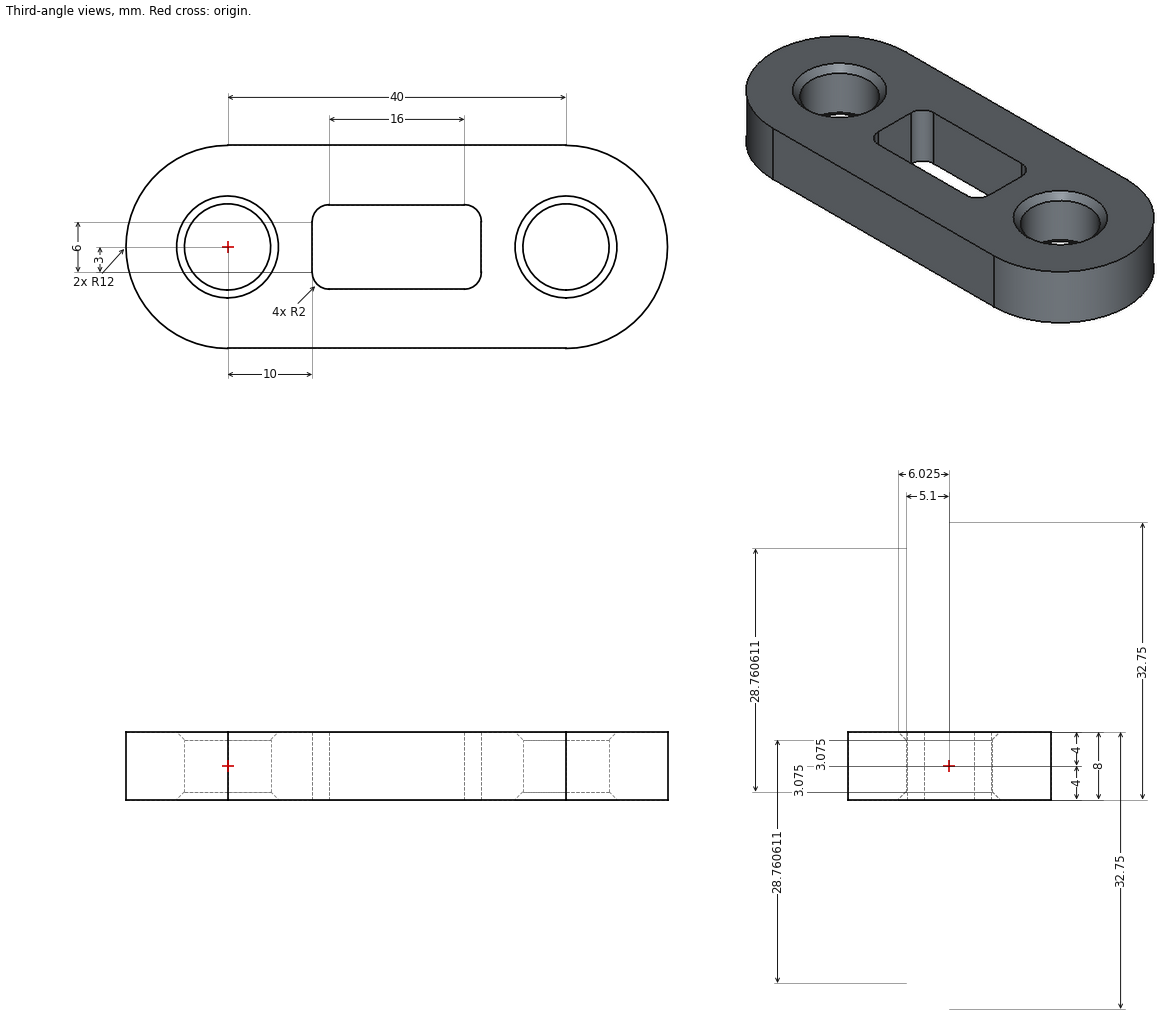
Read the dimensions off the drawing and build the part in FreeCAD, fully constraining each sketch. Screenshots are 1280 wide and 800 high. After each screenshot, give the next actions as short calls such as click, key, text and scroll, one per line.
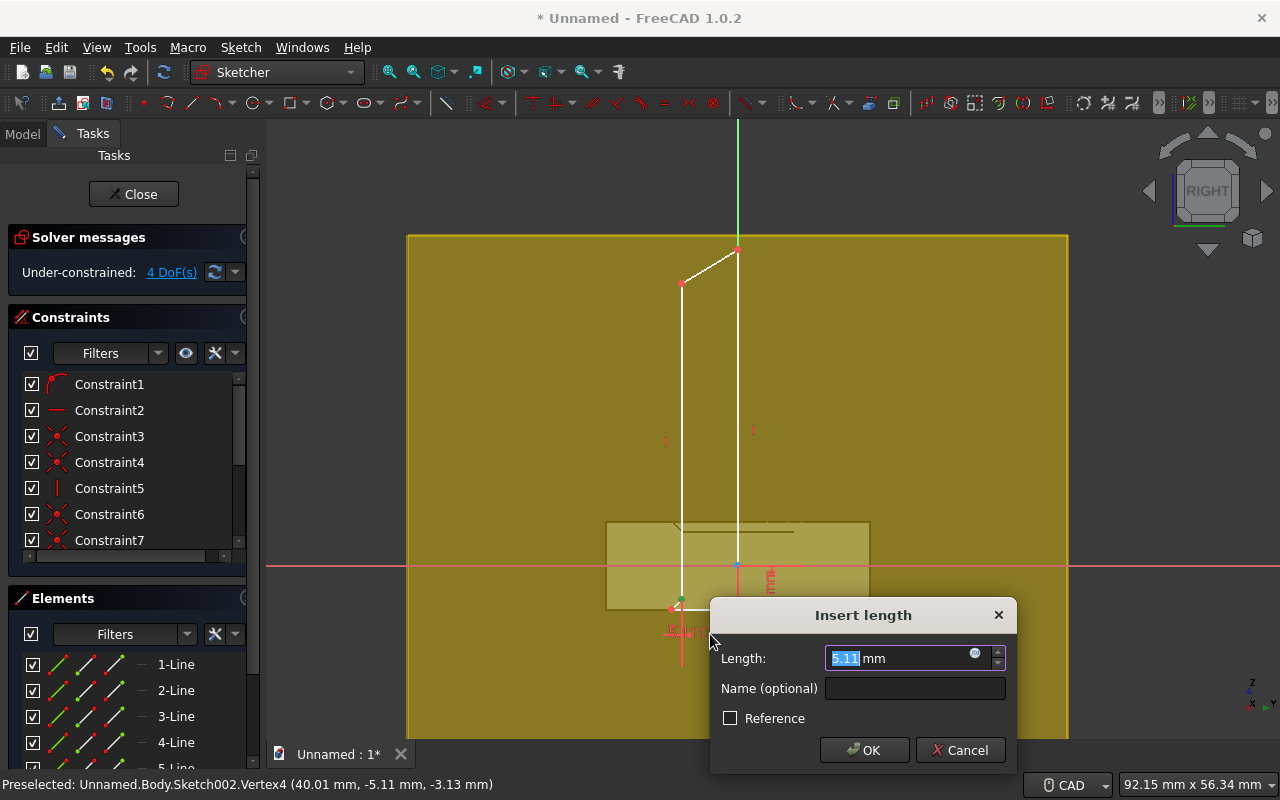
text(5.1)
key(Return)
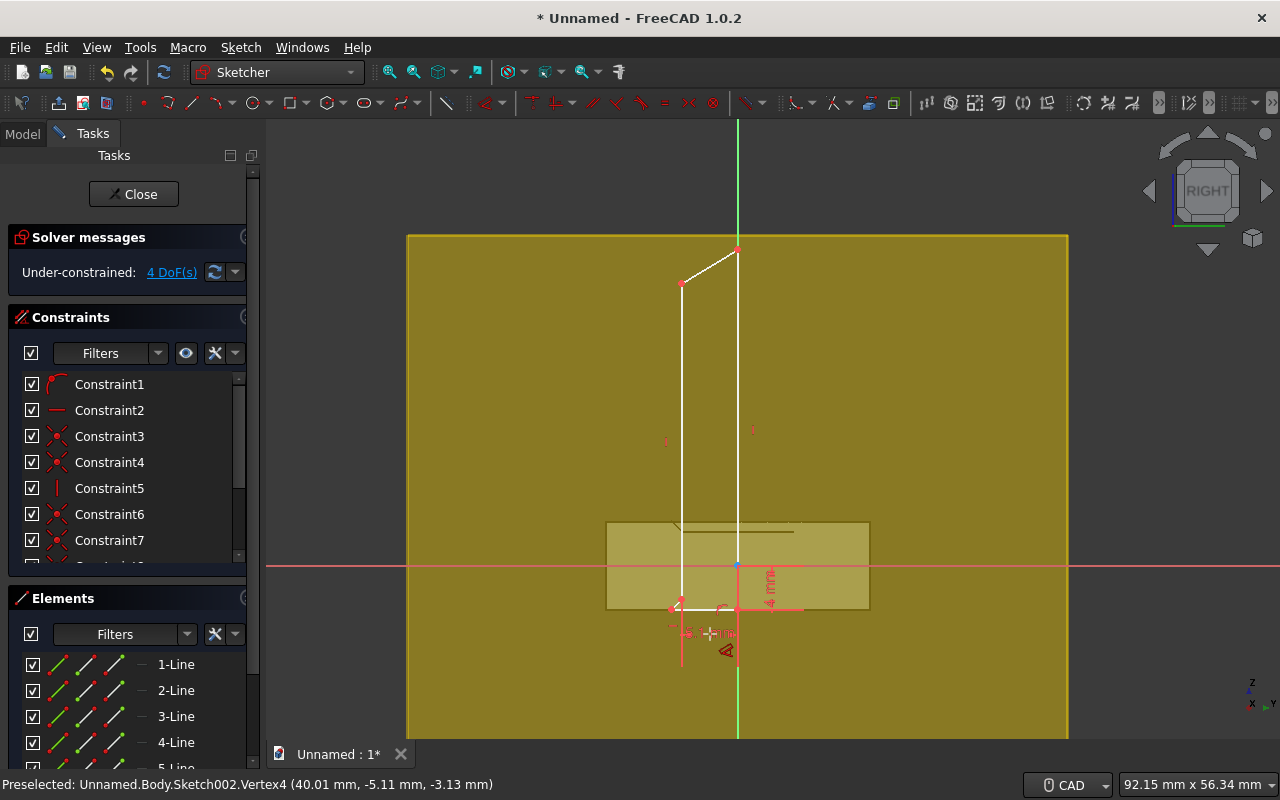
click(718, 610)
click(705, 668)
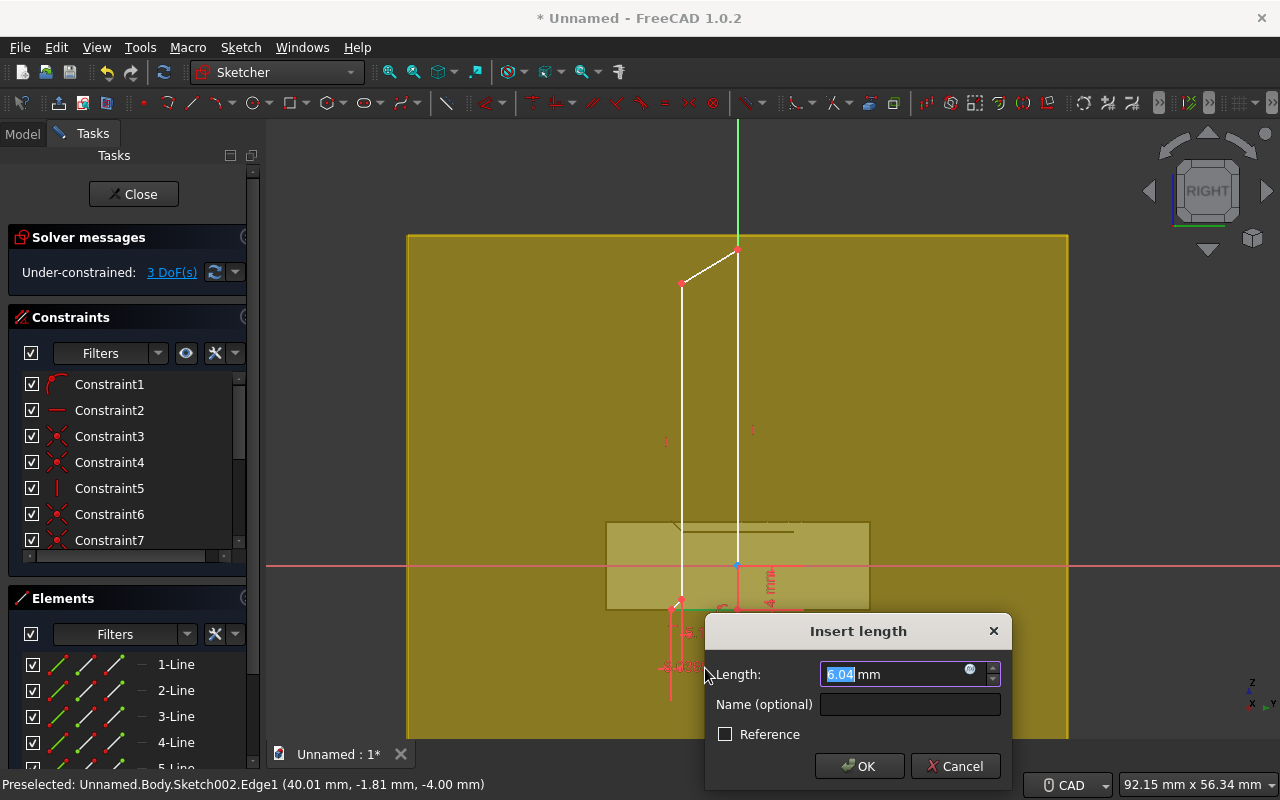
text(6.025)
key(Return)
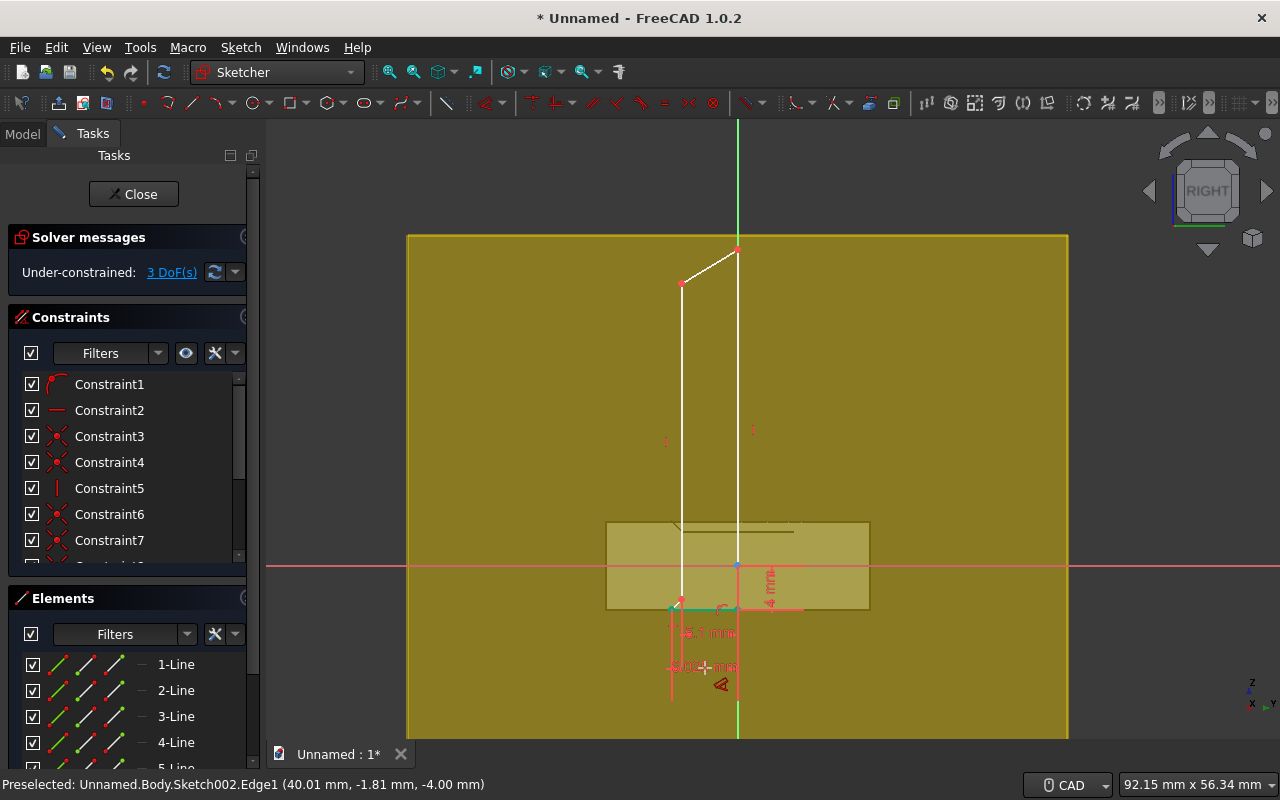
click(738, 358)
click(772, 430)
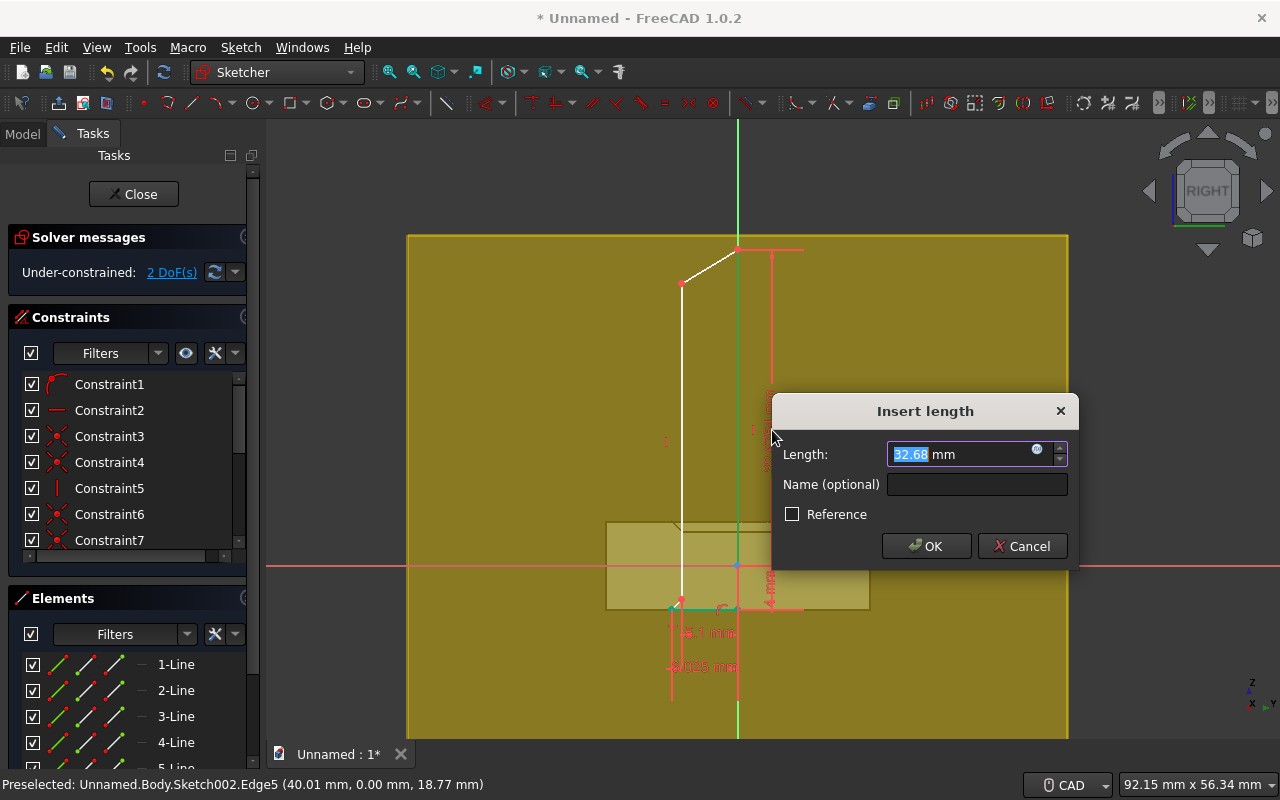
text(32.75)
key(Return)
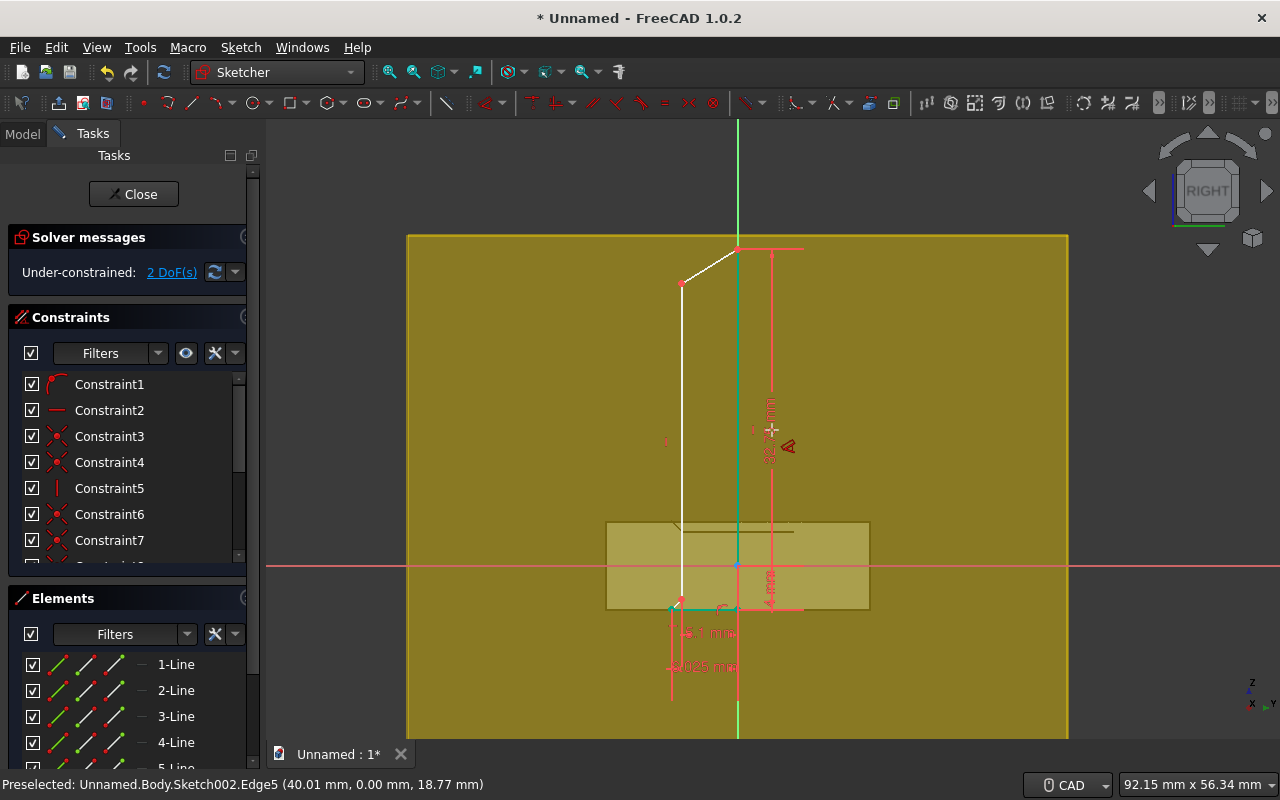
click(682, 600)
click(648, 583)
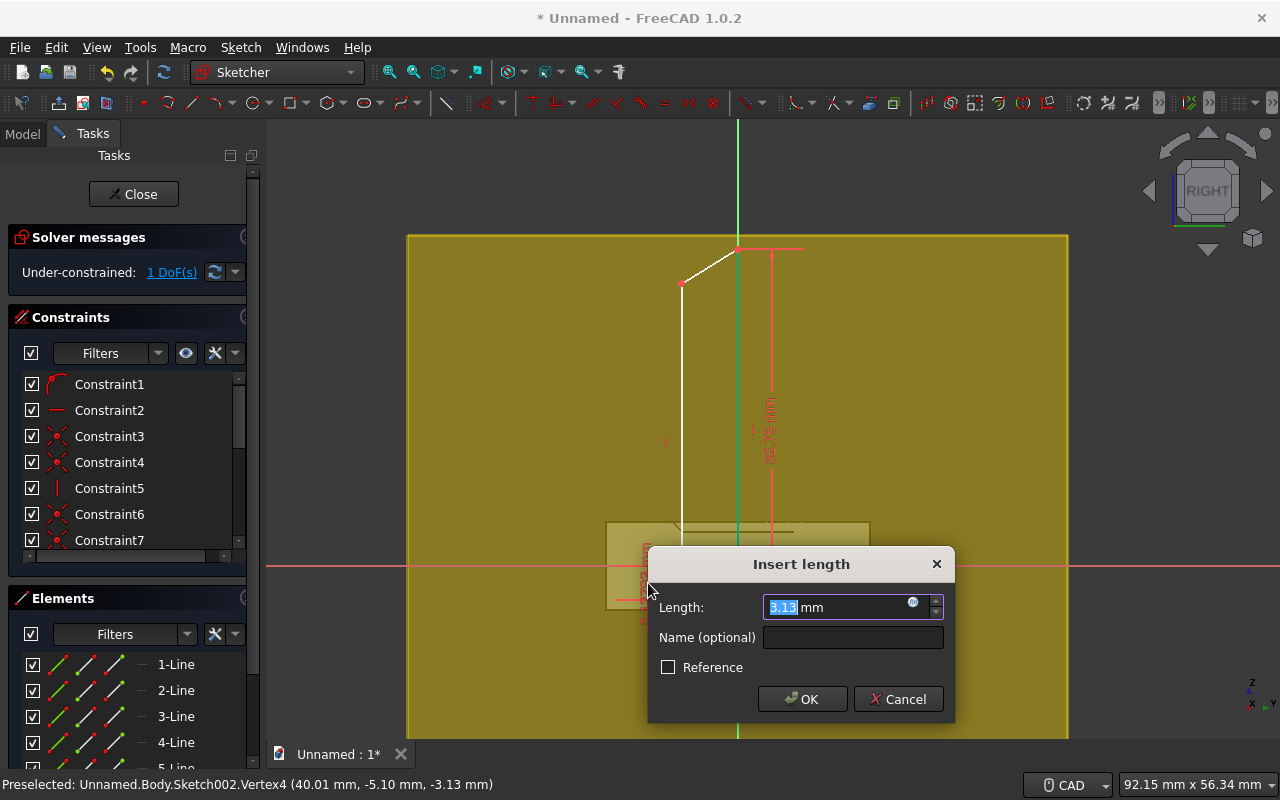
text(3.075)
key(Return)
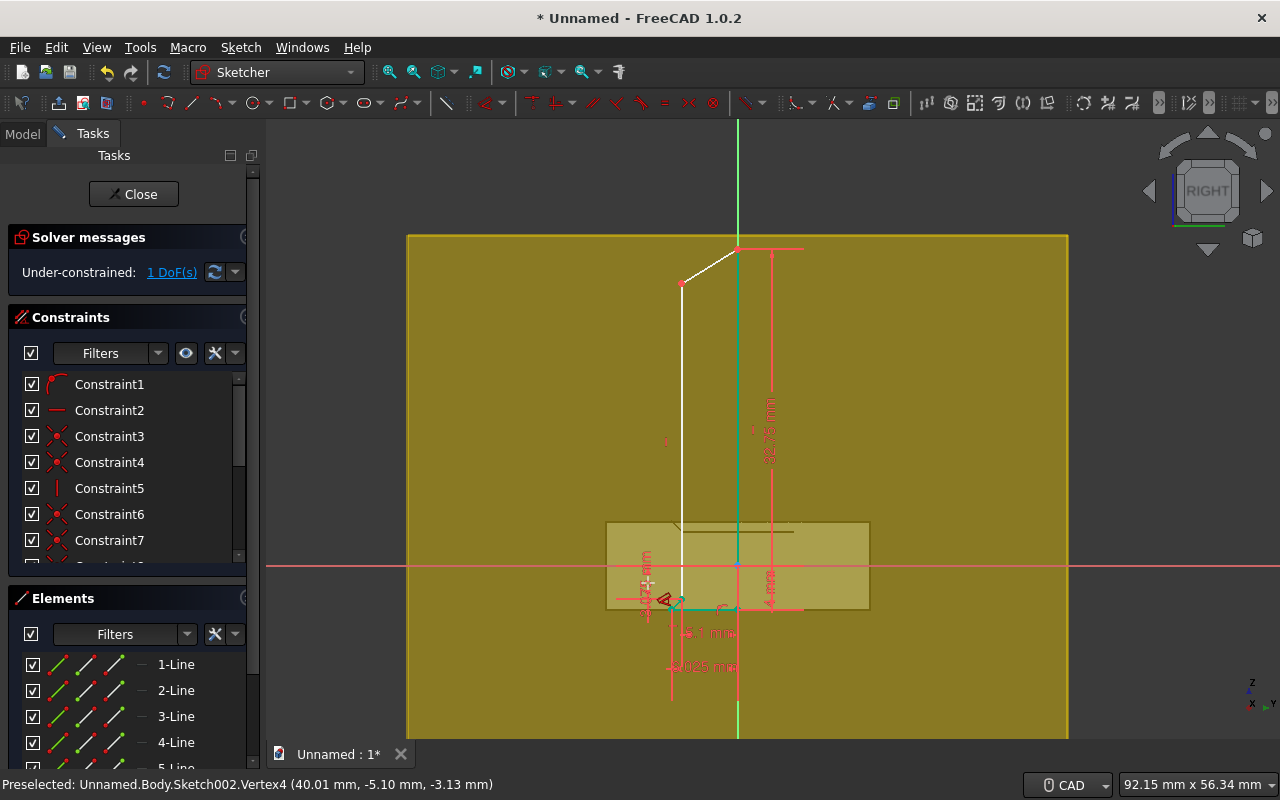
click(682, 505)
click(648, 442)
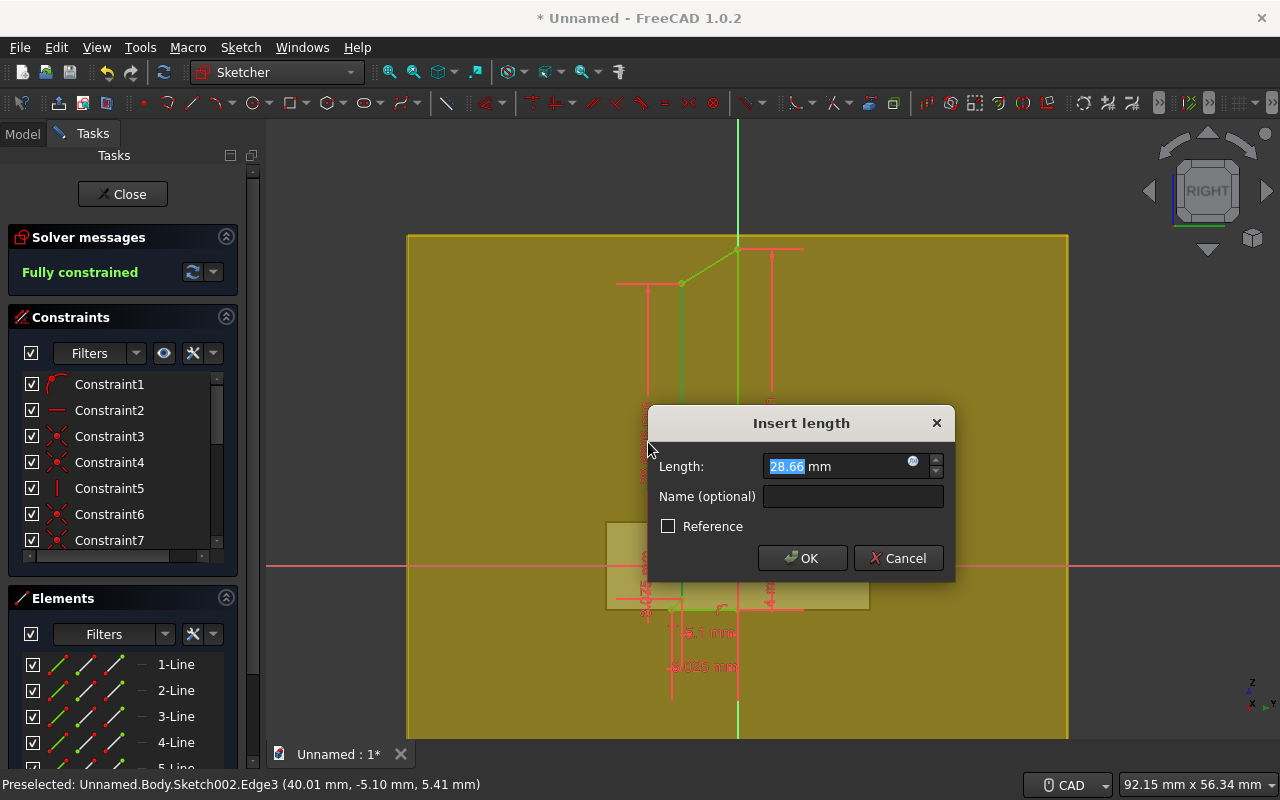
text(28.760611)
key(Return)
key(Escape)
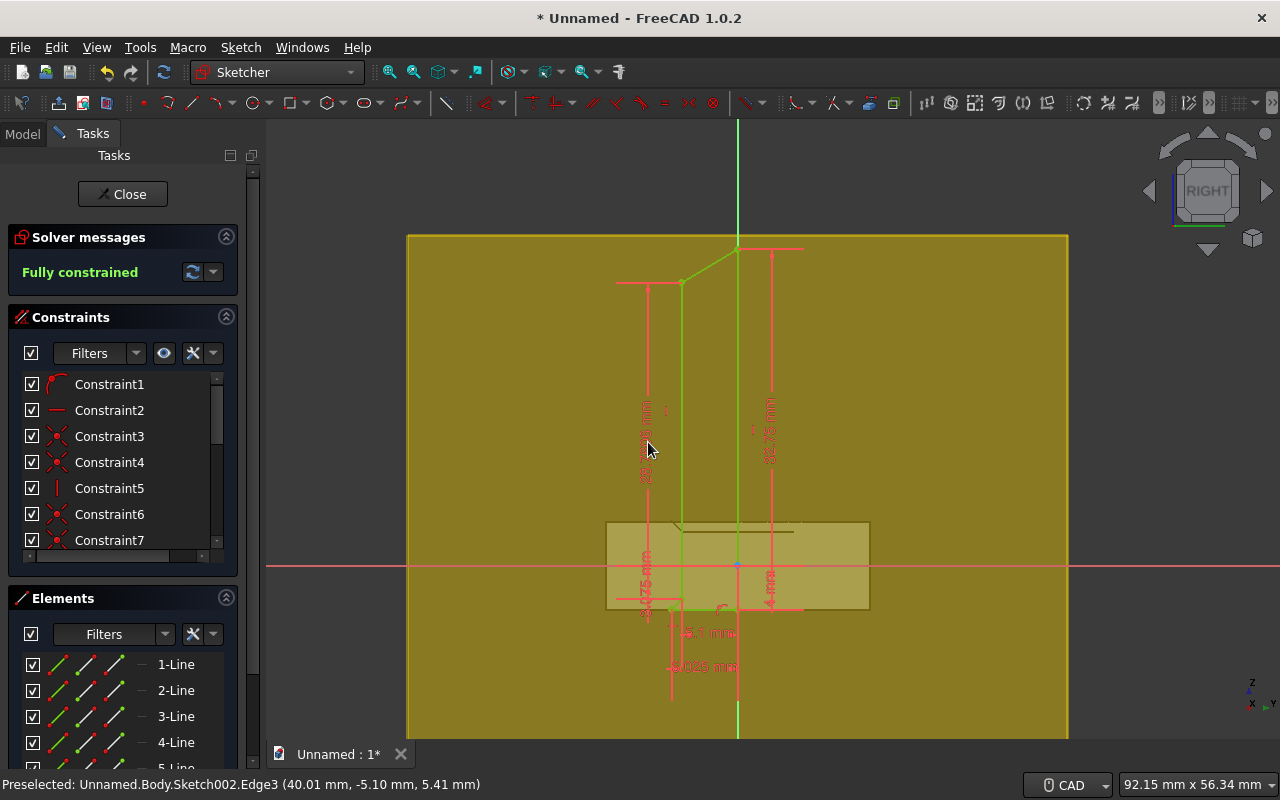
click(123, 194)